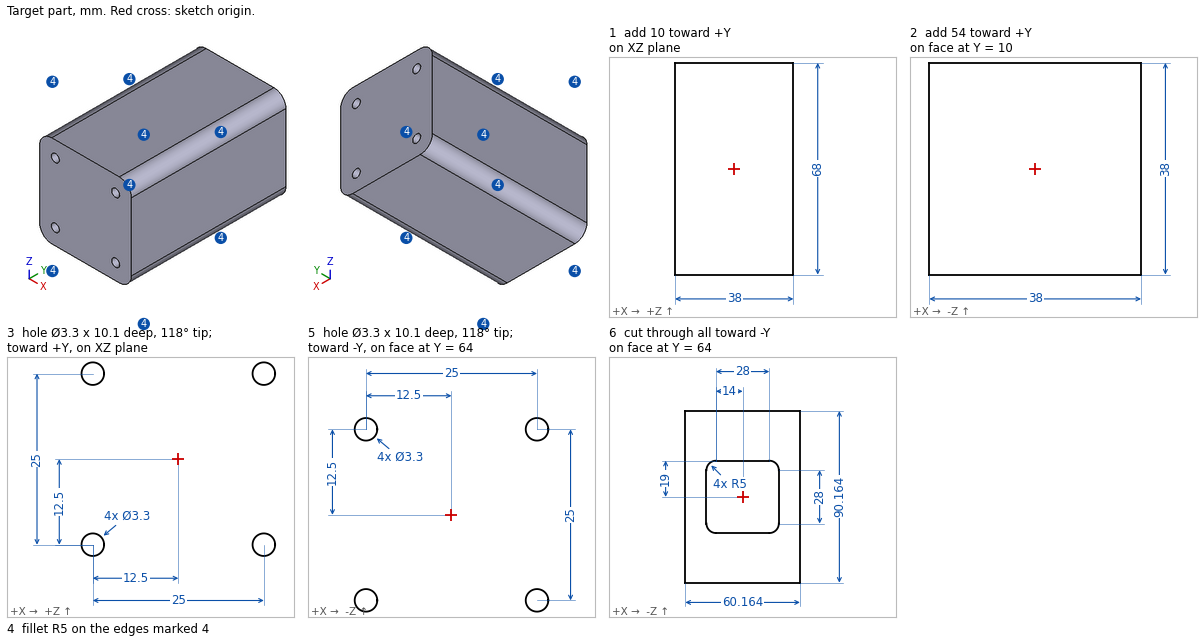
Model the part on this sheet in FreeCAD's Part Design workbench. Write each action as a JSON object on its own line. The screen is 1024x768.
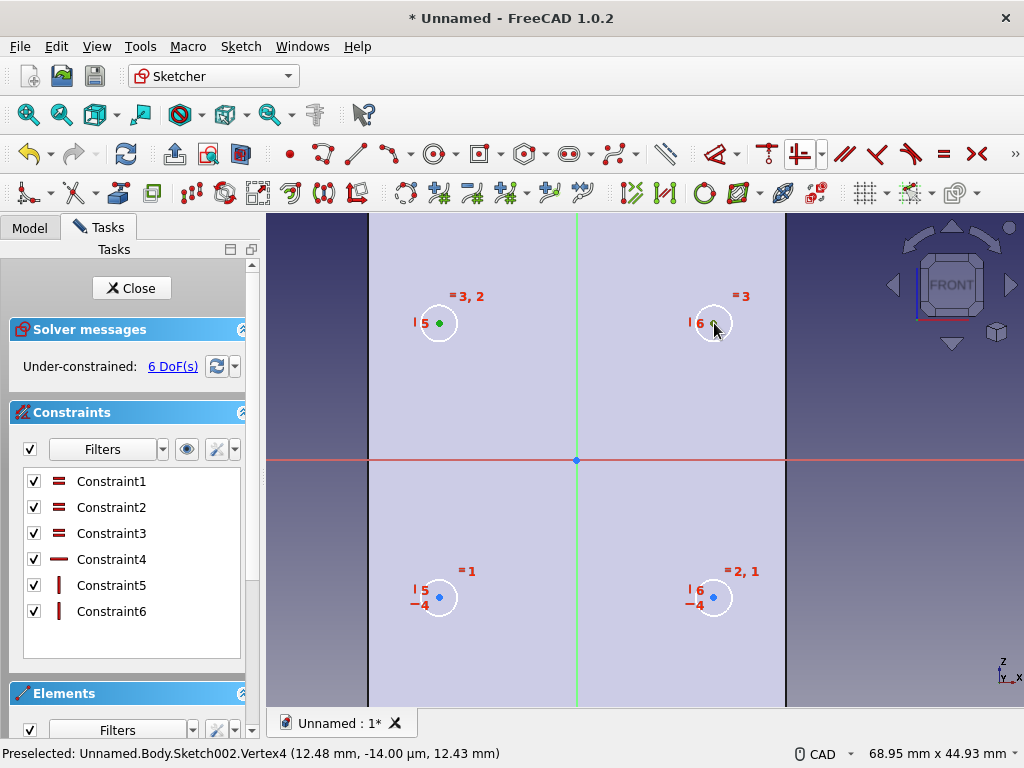
{"action": "left_click", "coordinate": [822, 154]}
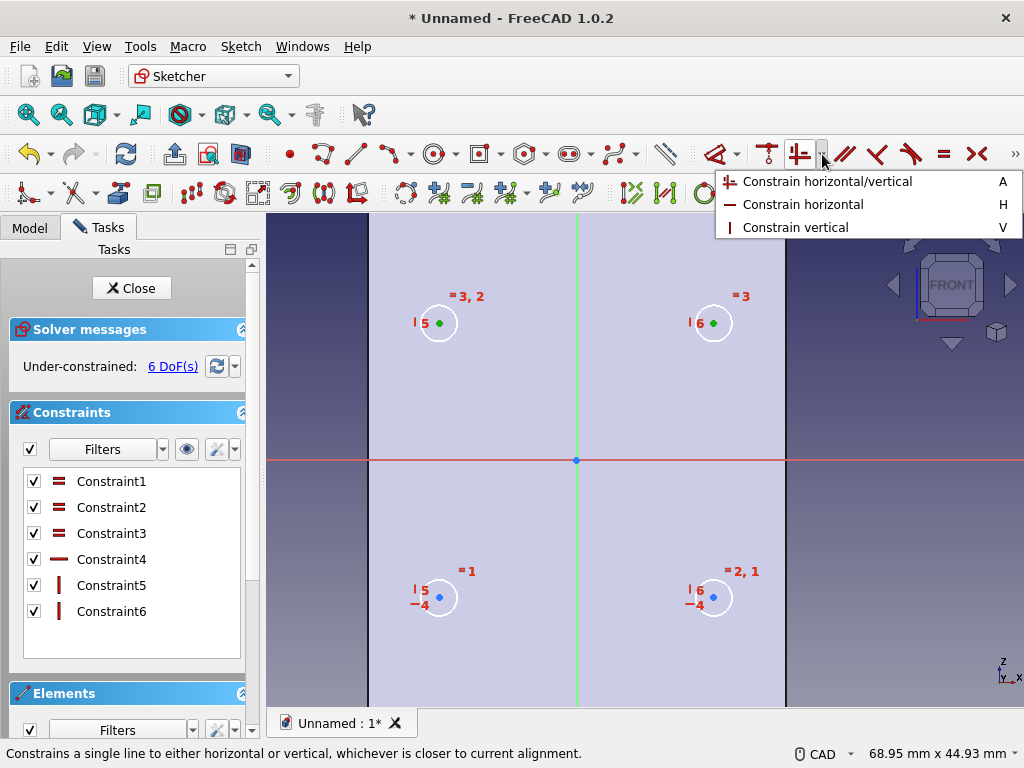
{"action": "left_click", "coordinate": [869, 204]}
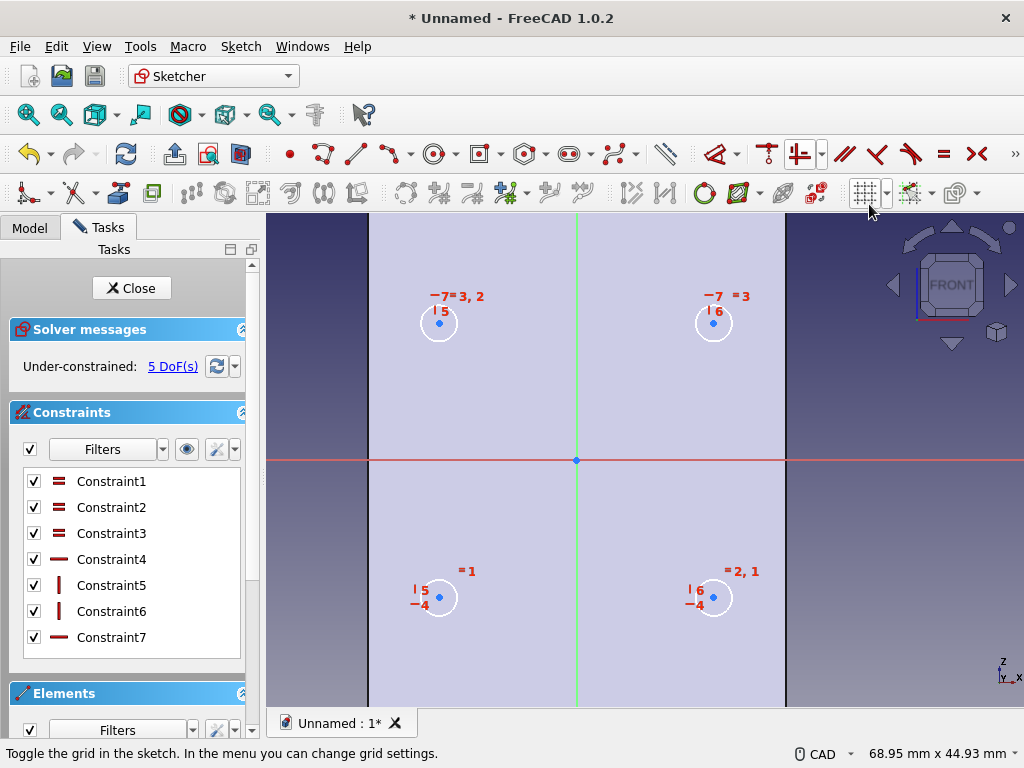
{"action": "left_click", "coordinate": [714, 154]}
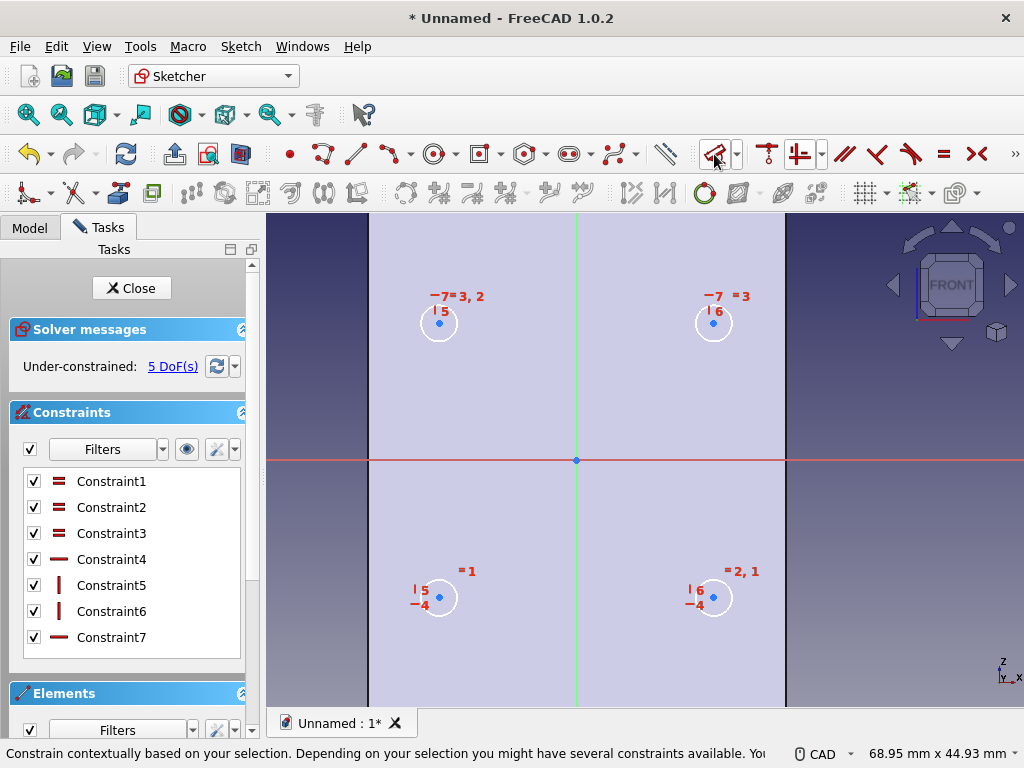
{"action": "left_click", "coordinate": [452, 585]}
{"action": "left_click", "coordinate": [475, 562]}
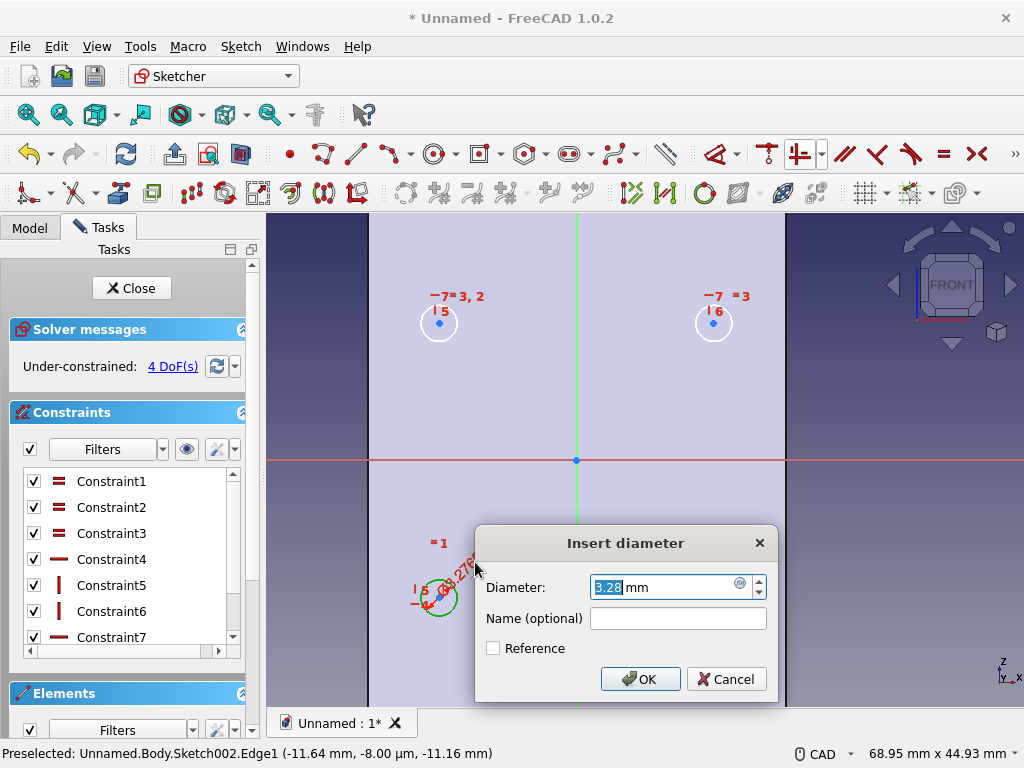
{"action": "type", "text": "3.3"}
{"action": "key", "text": "Return"}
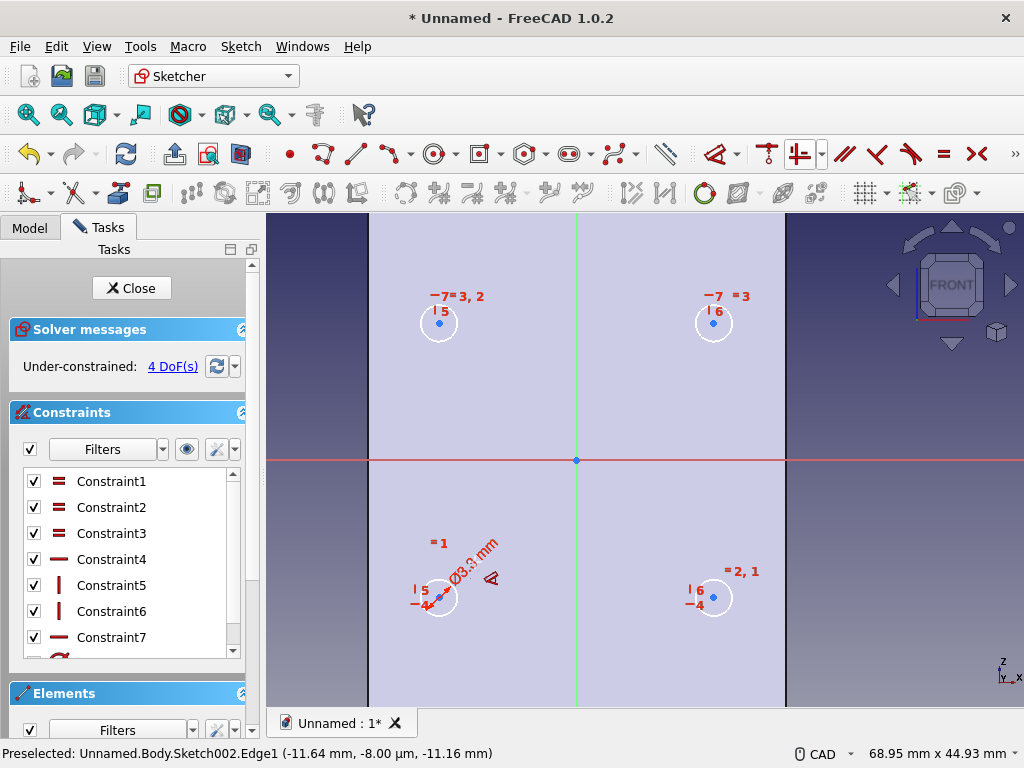
{"action": "left_click", "coordinate": [439, 598]}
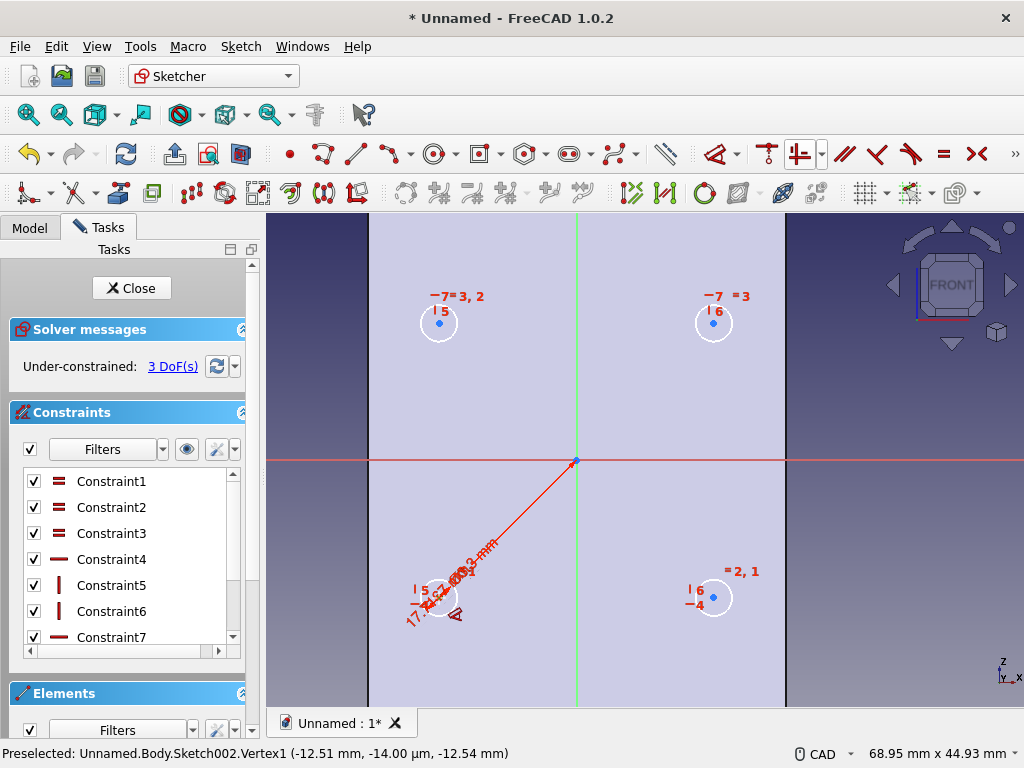
{"action": "left_click", "coordinate": [714, 598]}
{"action": "left_click", "coordinate": [513, 632]}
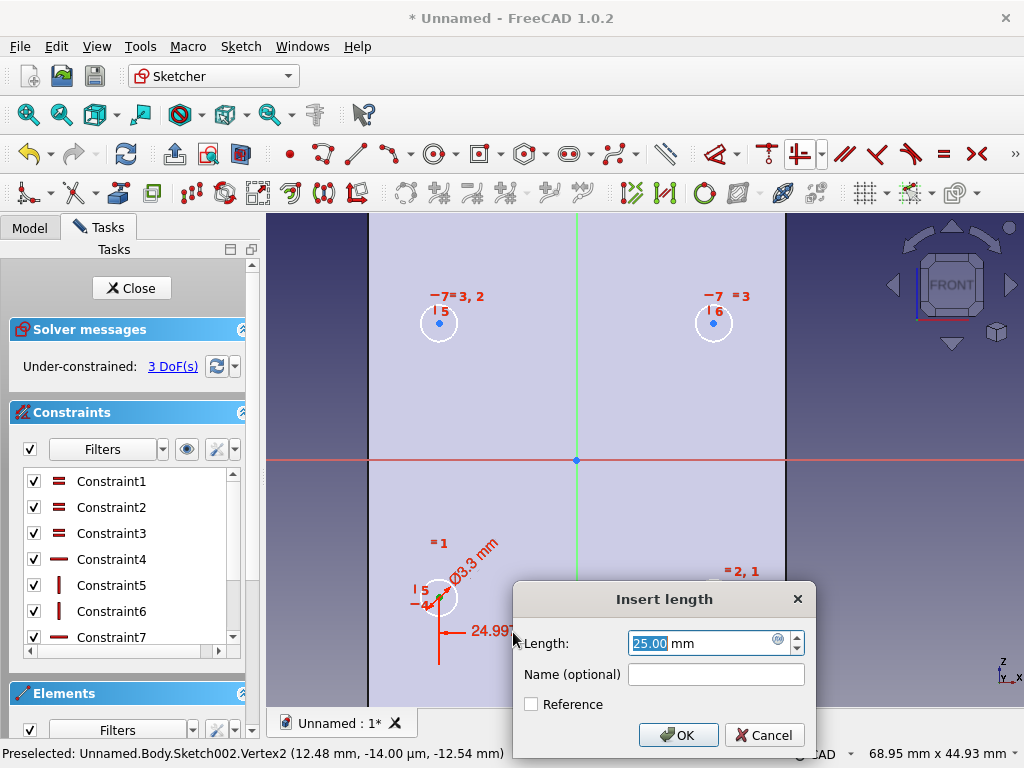
{"action": "type", "text": "25"}
{"action": "key", "text": "Return"}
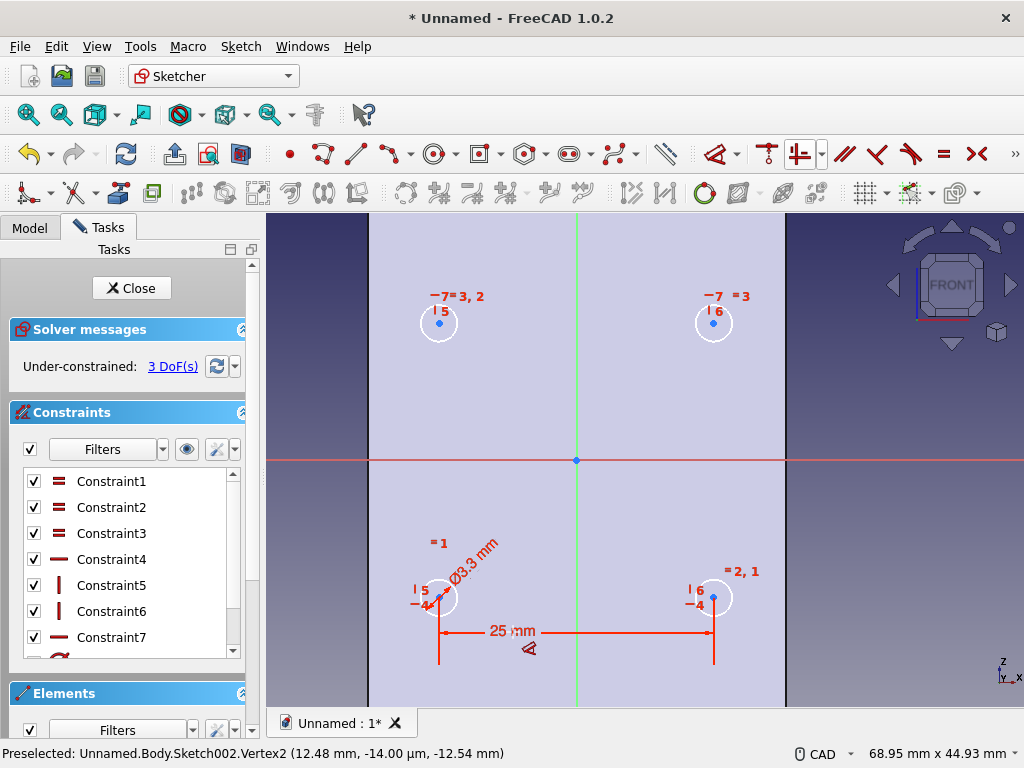
{"action": "left_click", "coordinate": [439, 598]}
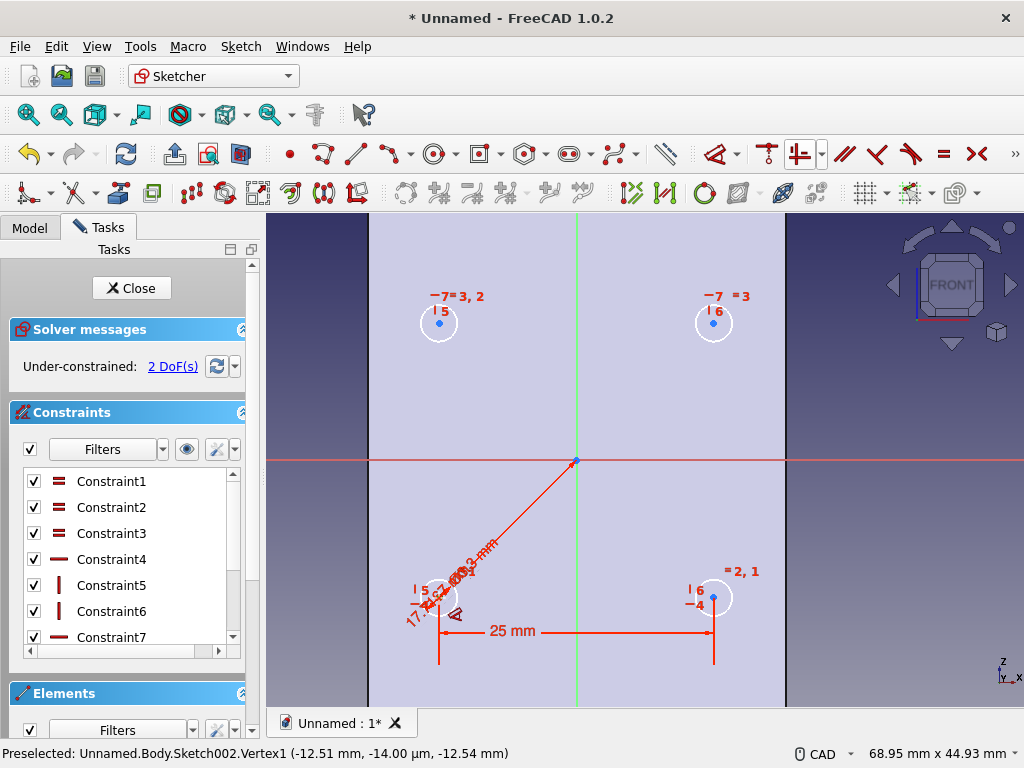
{"action": "left_click", "coordinate": [439, 323]}
{"action": "left_click", "coordinate": [405, 398]}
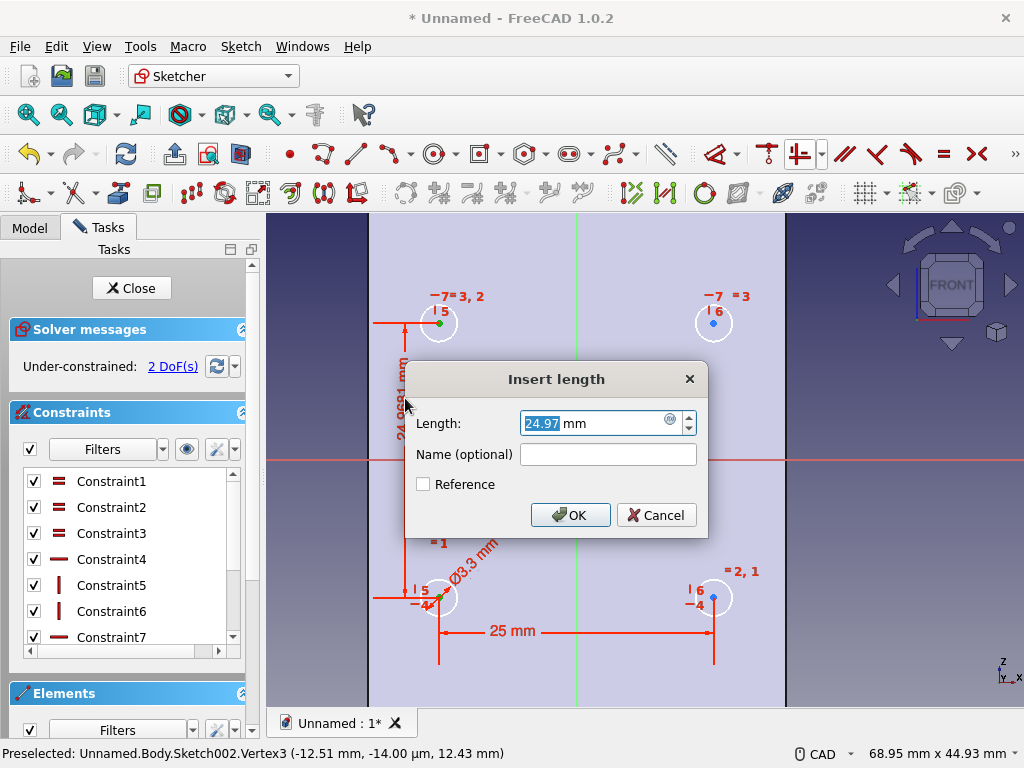
{"action": "type", "text": "25"}
{"action": "key", "text": "Return"}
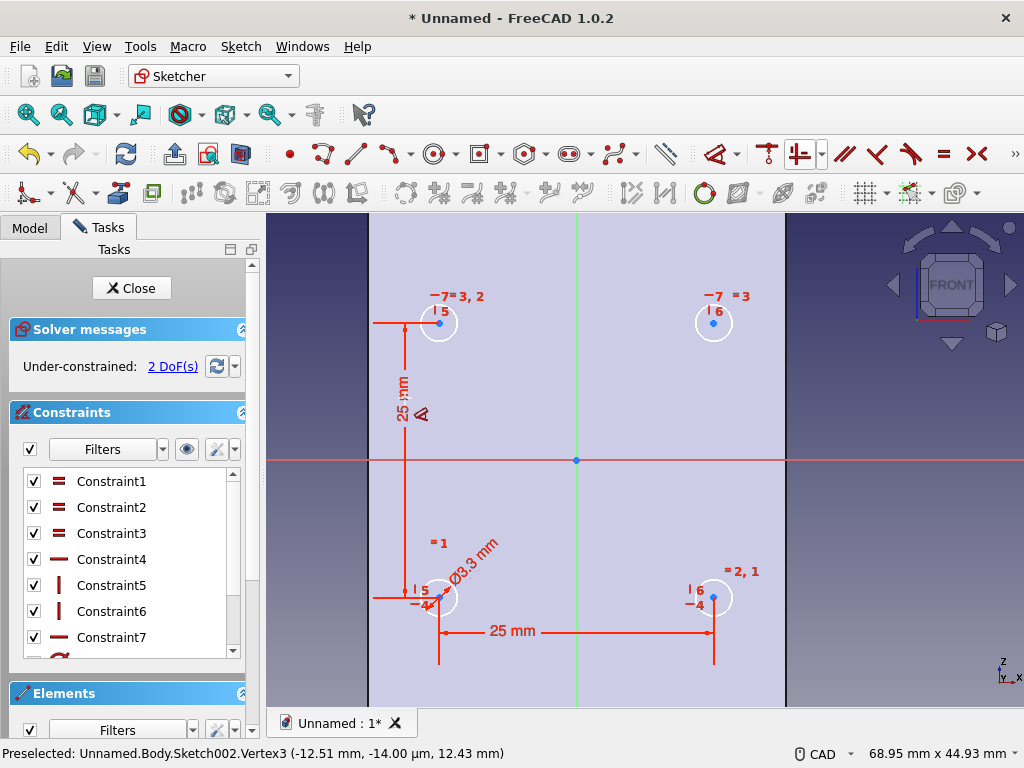
{"action": "left_click", "coordinate": [439, 598]}
{"action": "left_click", "coordinate": [508, 426]}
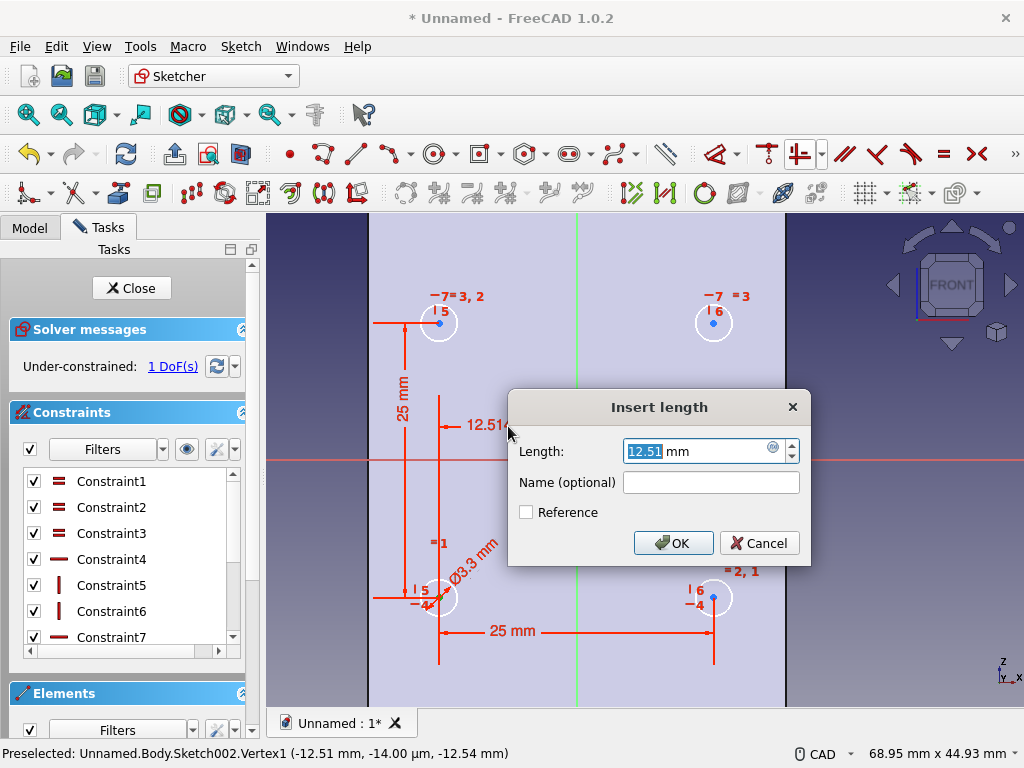
{"action": "type", "text": "12.5"}
{"action": "key", "text": "Return"}